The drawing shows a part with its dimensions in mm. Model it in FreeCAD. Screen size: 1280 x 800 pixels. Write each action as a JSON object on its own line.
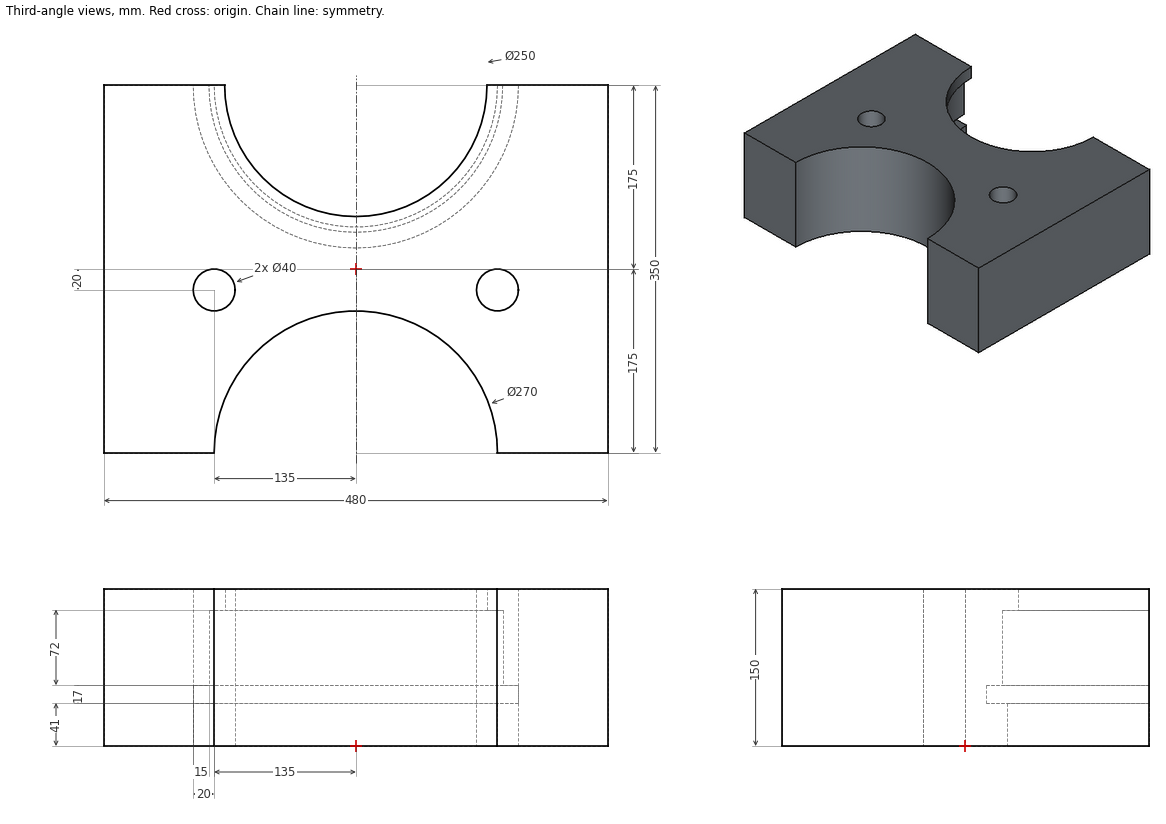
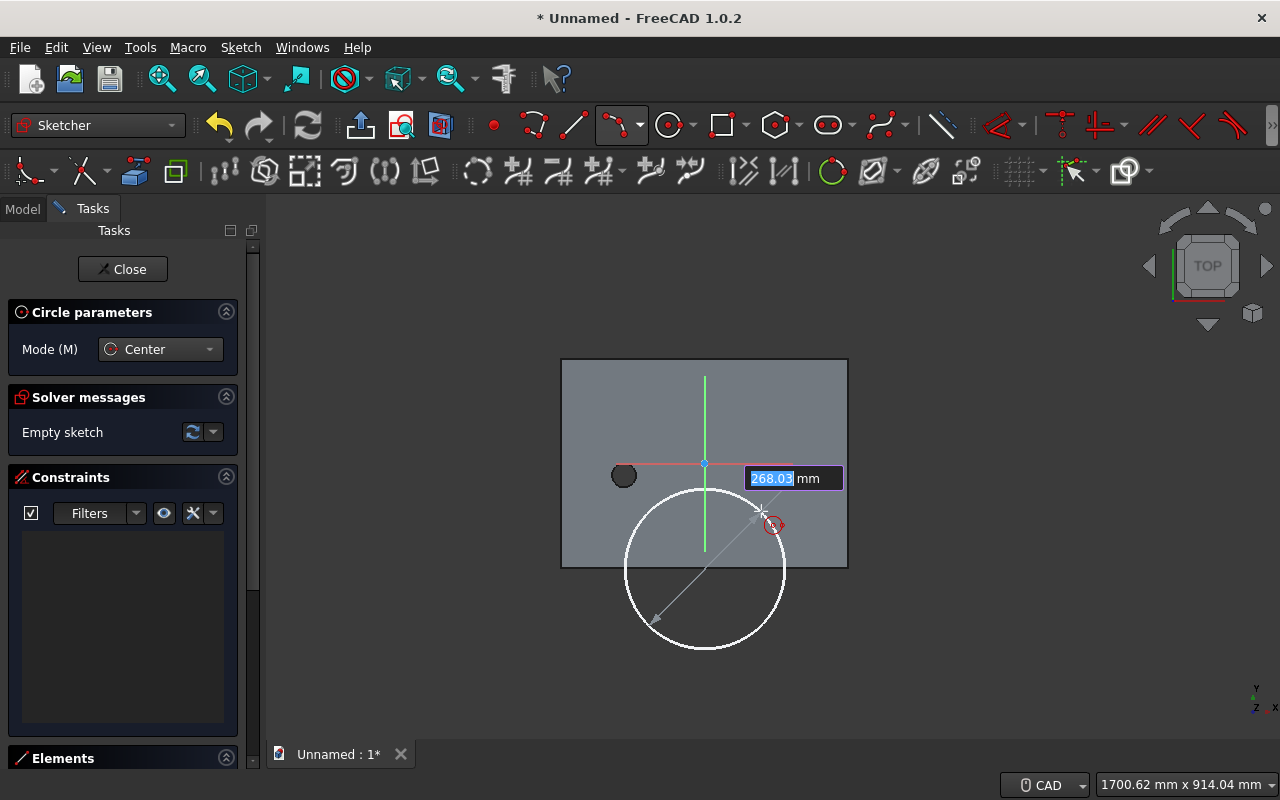
{"action": "type", "text": "270"}
{"action": "key", "text": "Return"}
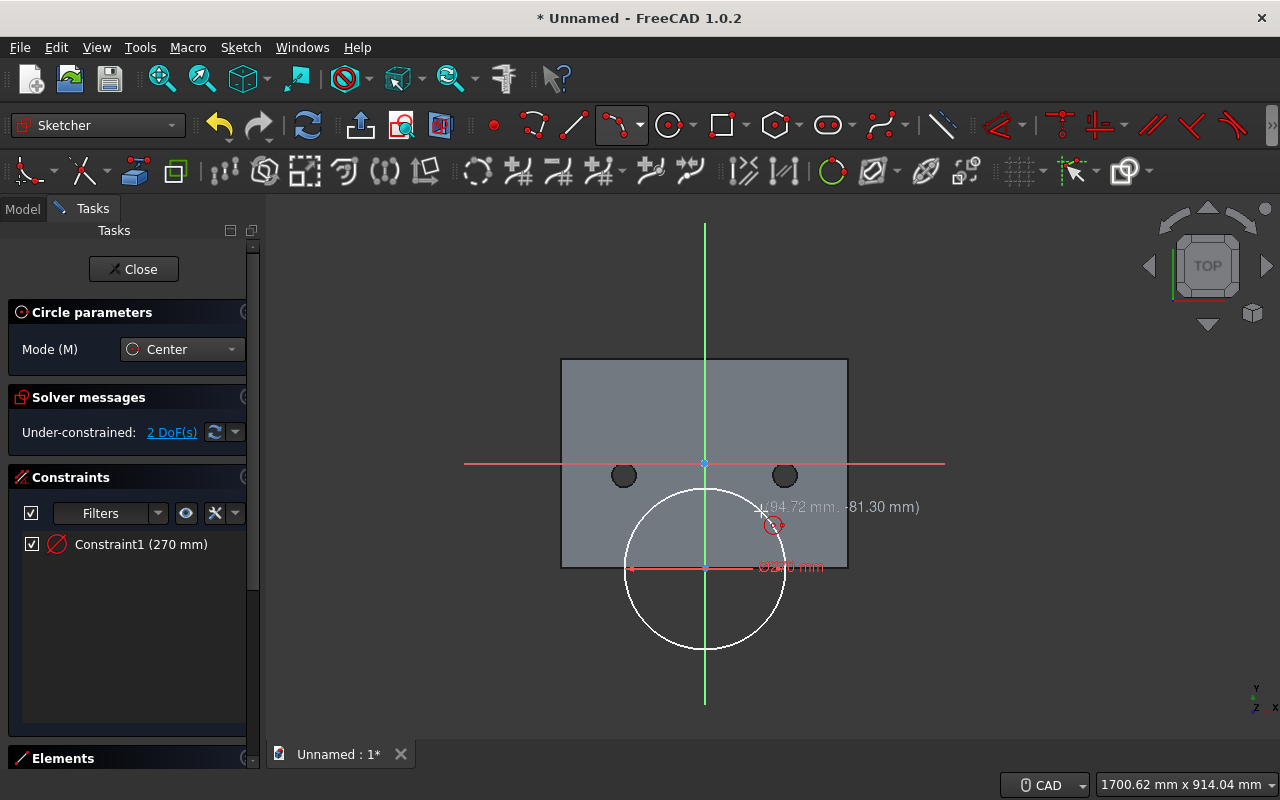
{"action": "left_click", "coordinate": [705, 359]}
{"action": "mouse_move", "coordinate": [757, 306]}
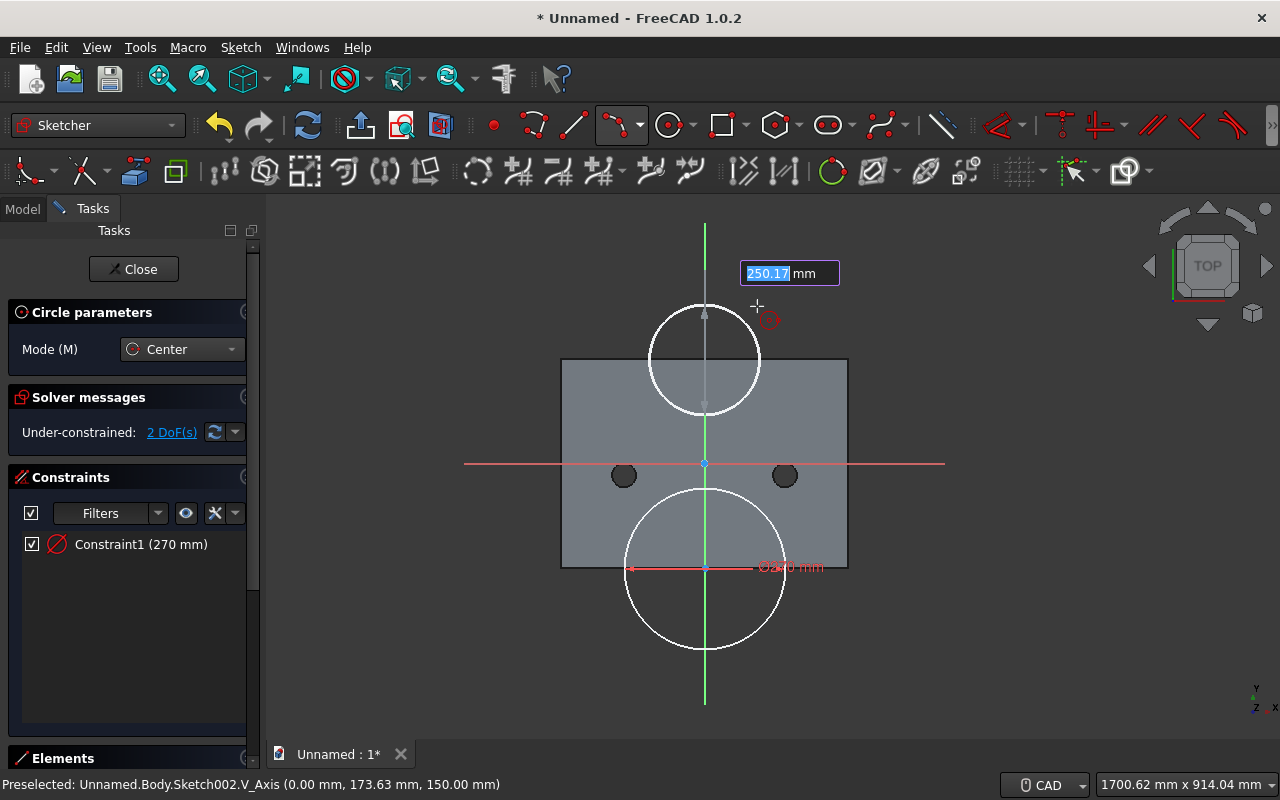
{"action": "type", "text": "250"}
{"action": "key", "text": "Return"}
{"action": "key", "text": "Escape"}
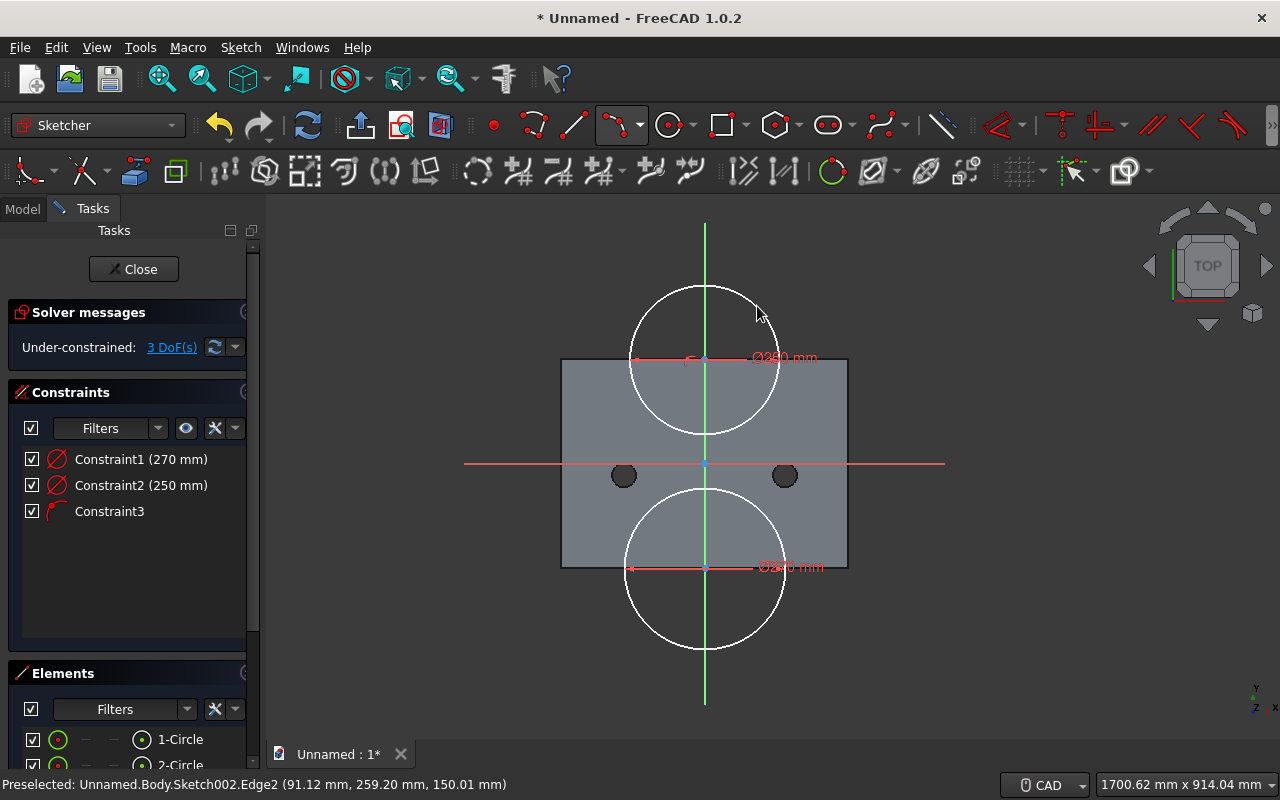
{"action": "left_click", "coordinate": [705, 569]}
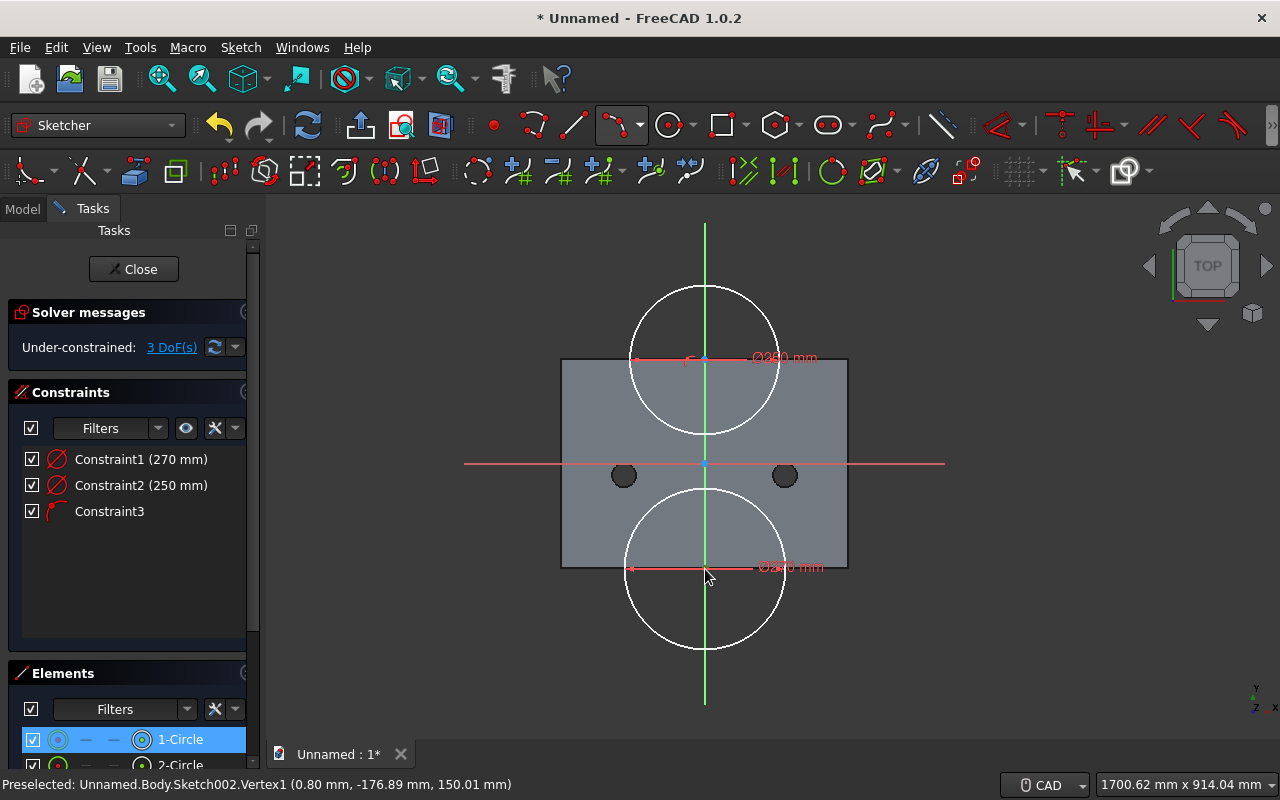
{"action": "left_click", "coordinate": [705, 606]}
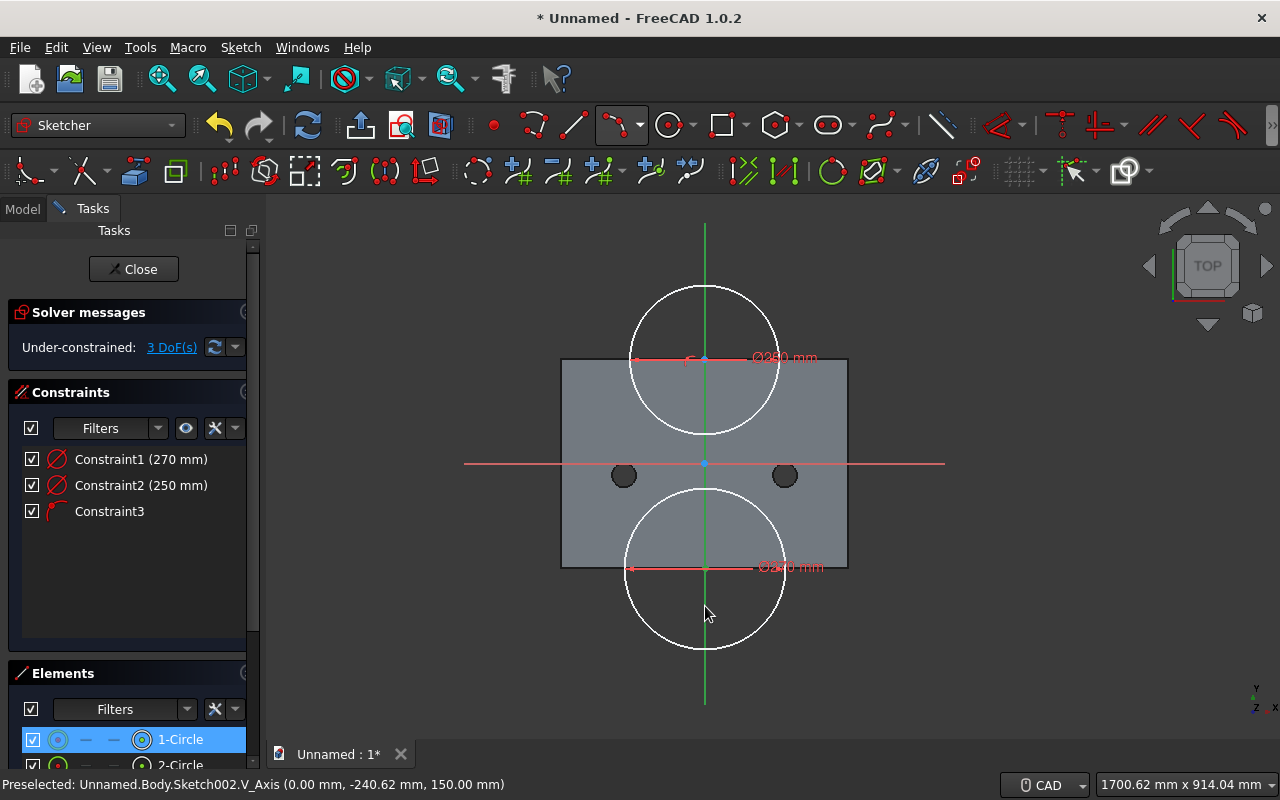
{"action": "key", "text": "c"}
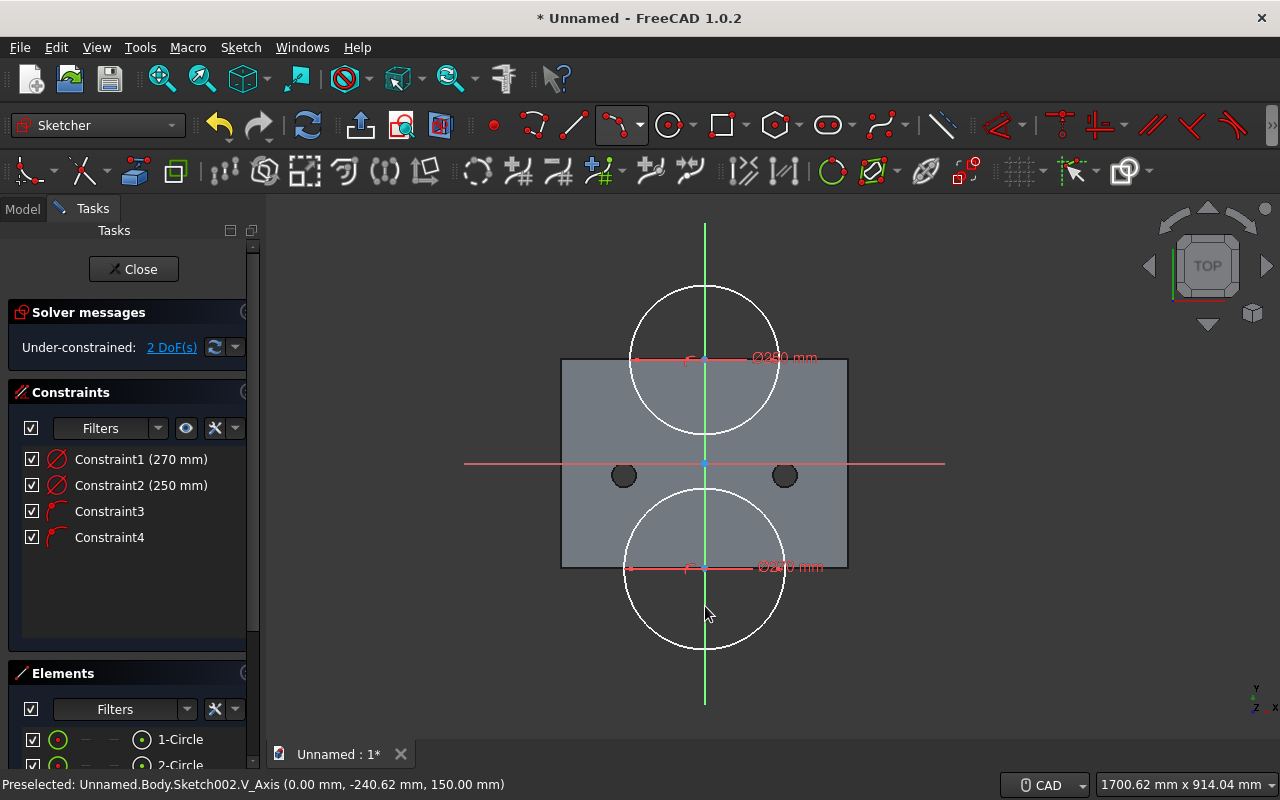
{"action": "key", "text": "d"}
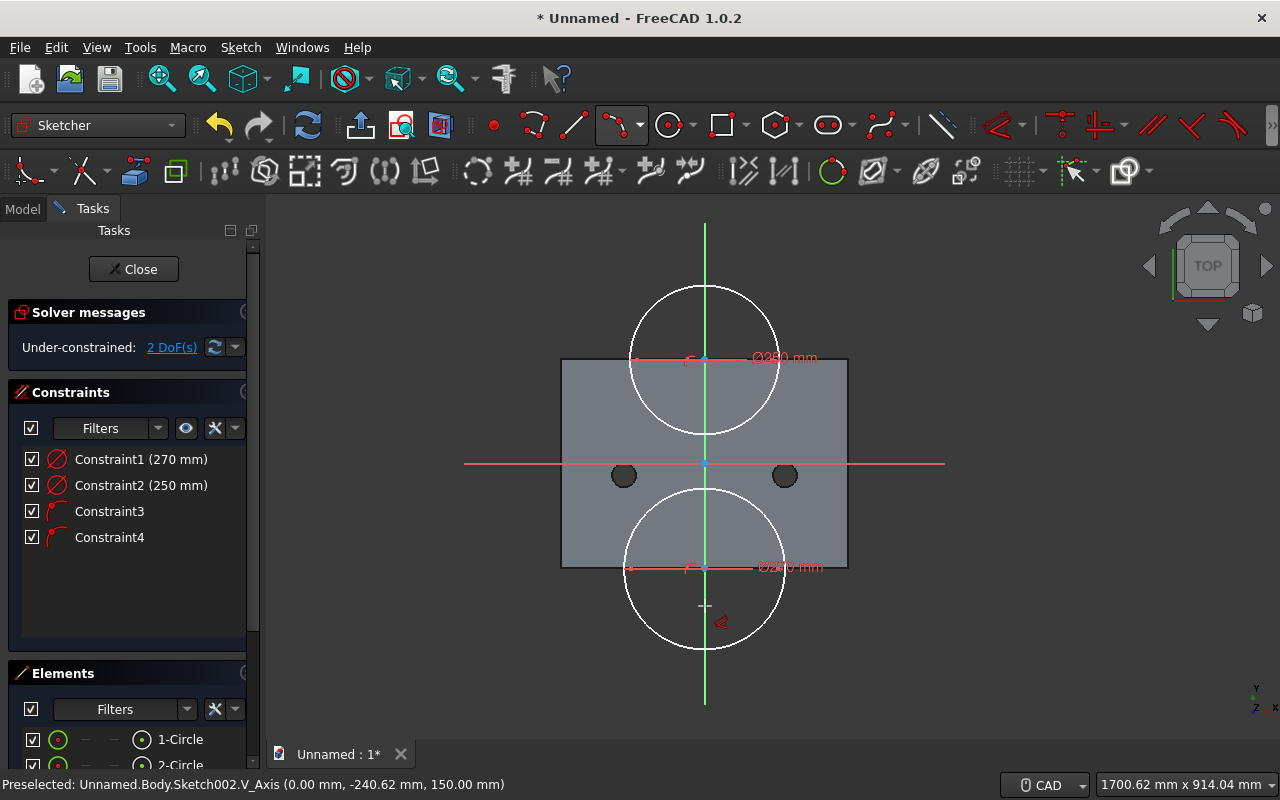
{"action": "left_click", "coordinate": [705, 569]}
{"action": "left_click", "coordinate": [739, 516]}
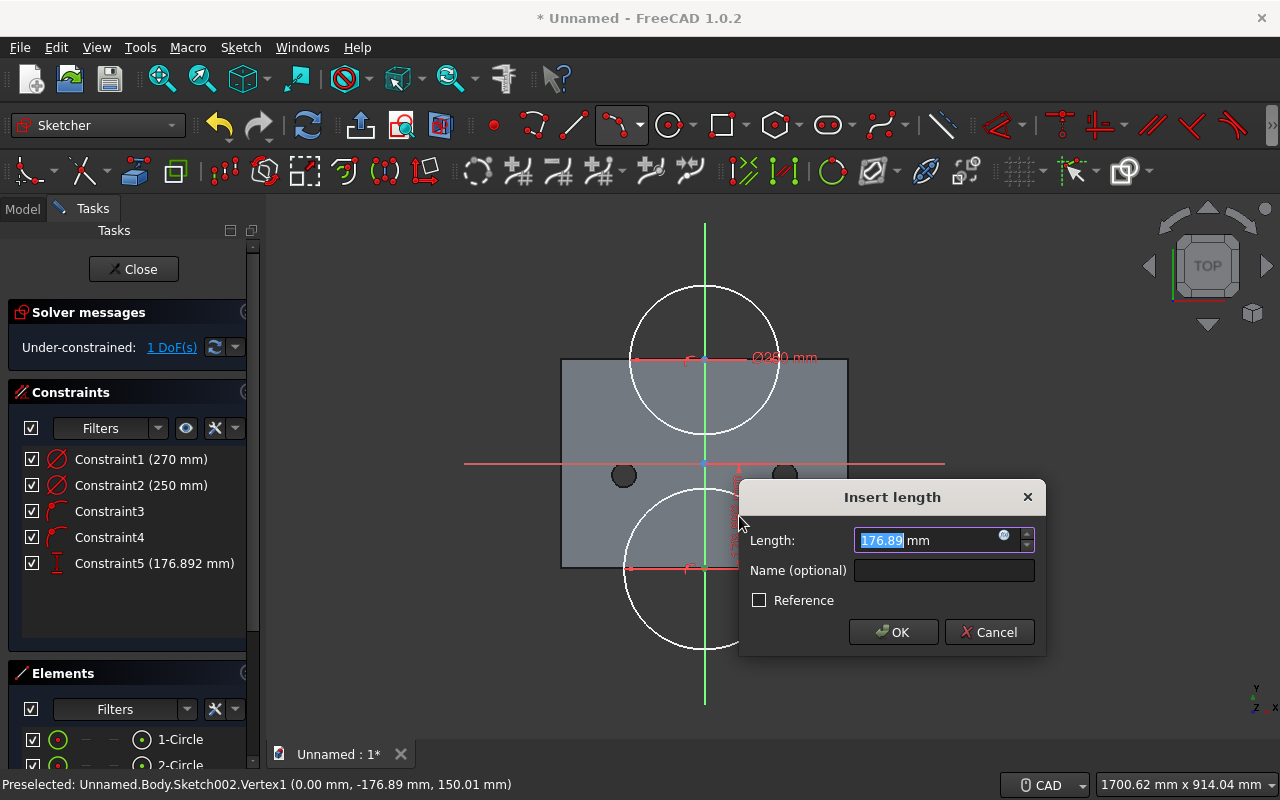
{"action": "type", "text": "175"}
{"action": "key", "text": "Return"}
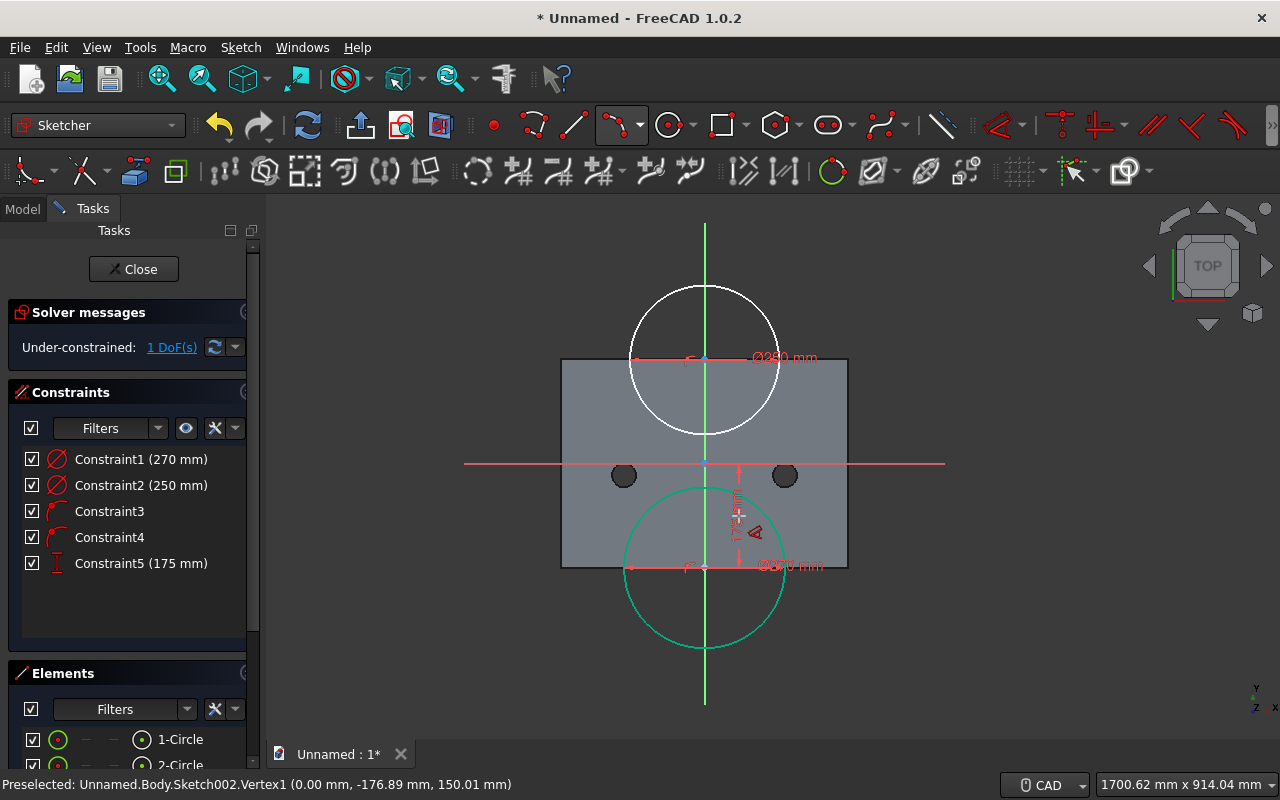
{"action": "left_click", "coordinate": [705, 360]}
{"action": "left_click", "coordinate": [739, 388]}